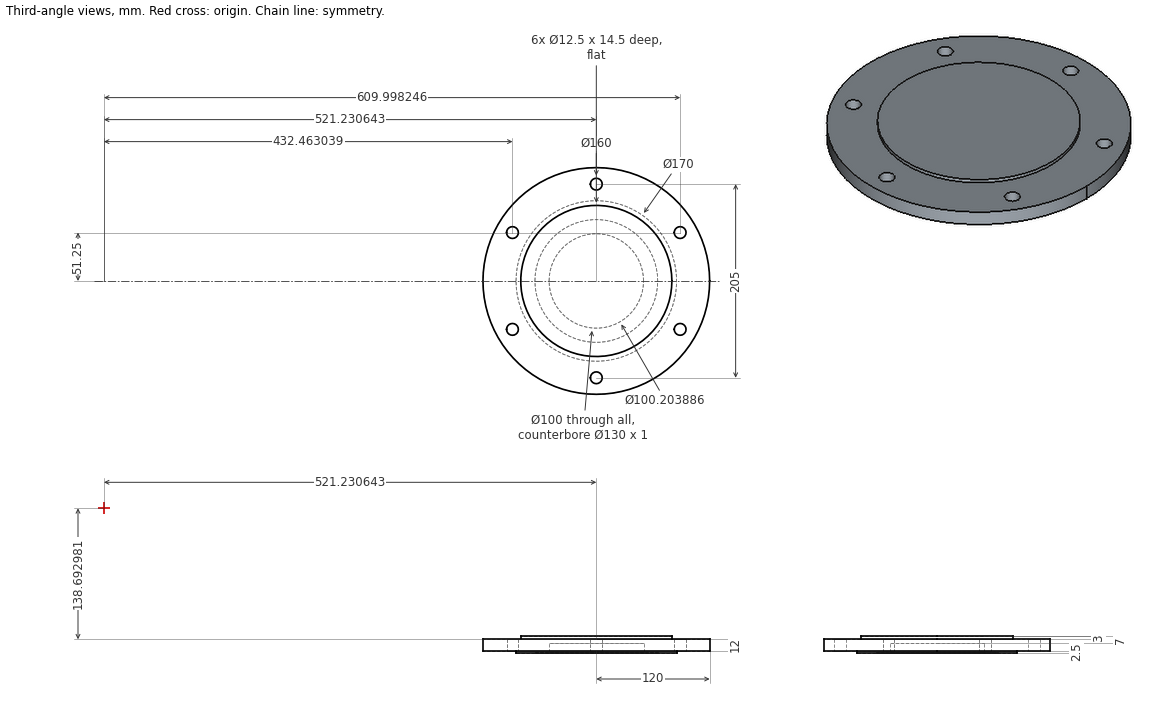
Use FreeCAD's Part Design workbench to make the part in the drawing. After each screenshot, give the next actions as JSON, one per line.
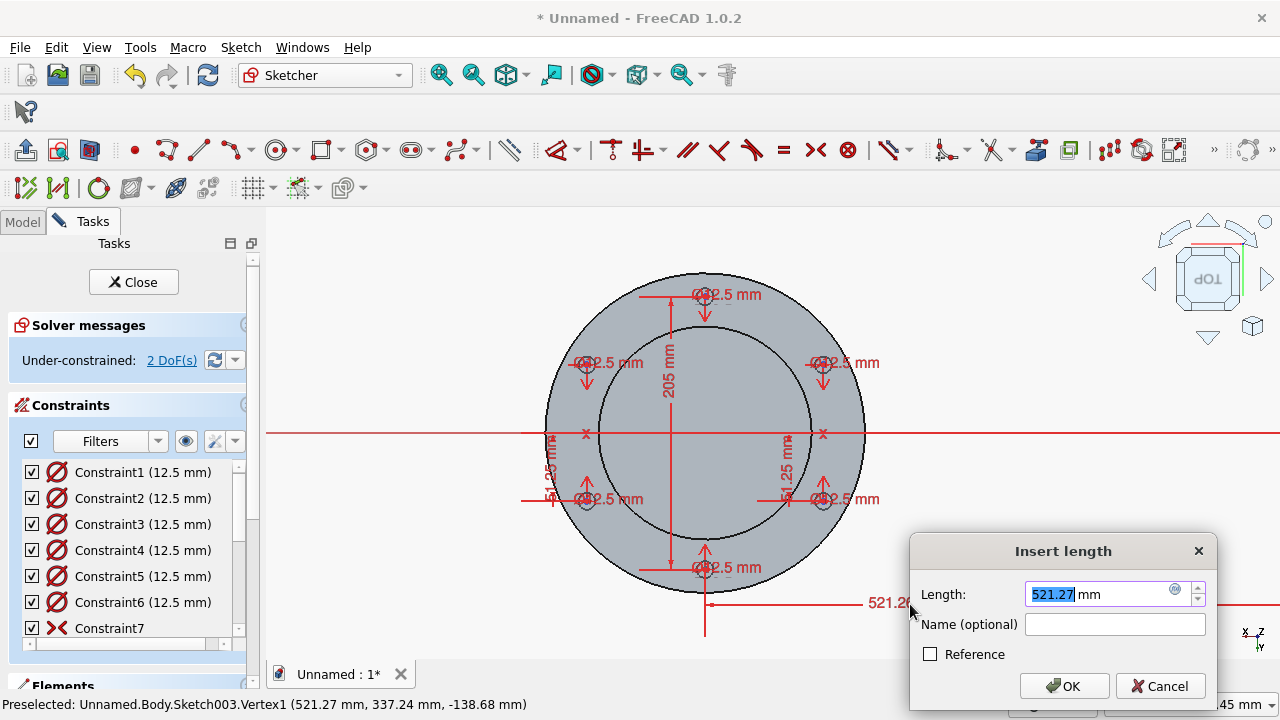
{"action": "type", "text": "521.230643"}
{"action": "key", "text": "Return"}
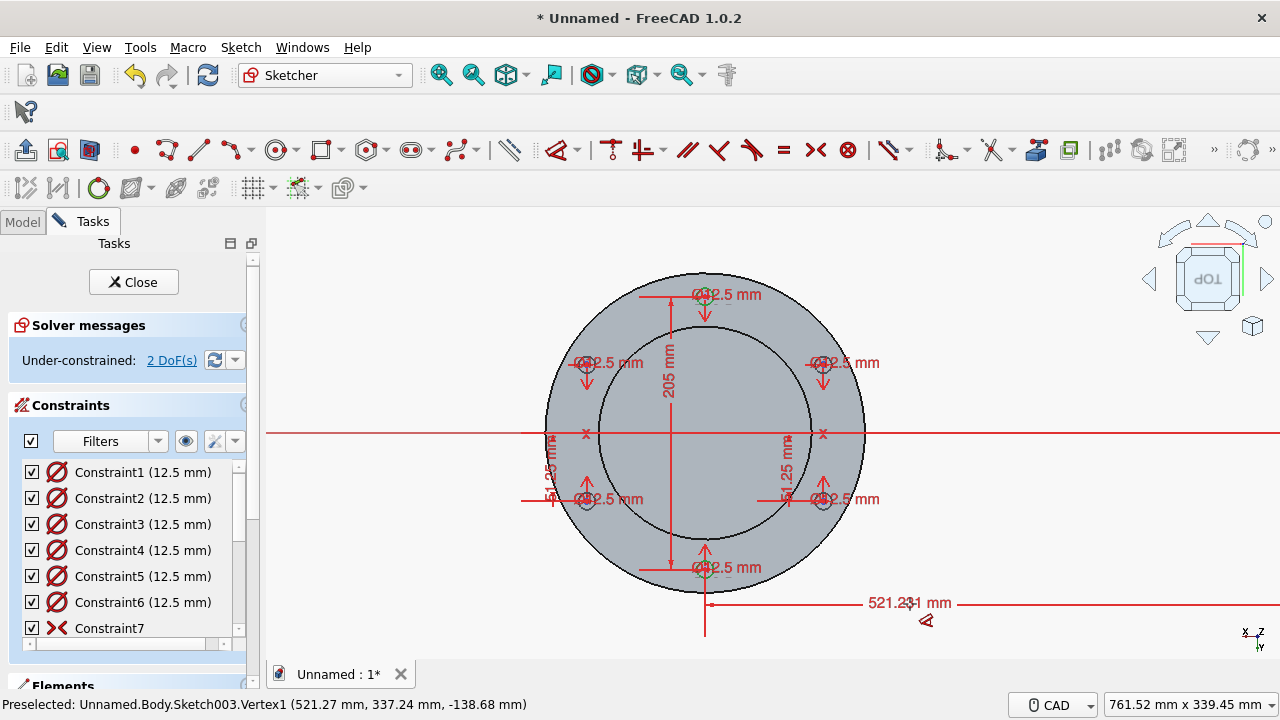
{"action": "left_click", "coordinate": [587, 501]}
{"action": "left_click", "coordinate": [851, 535]}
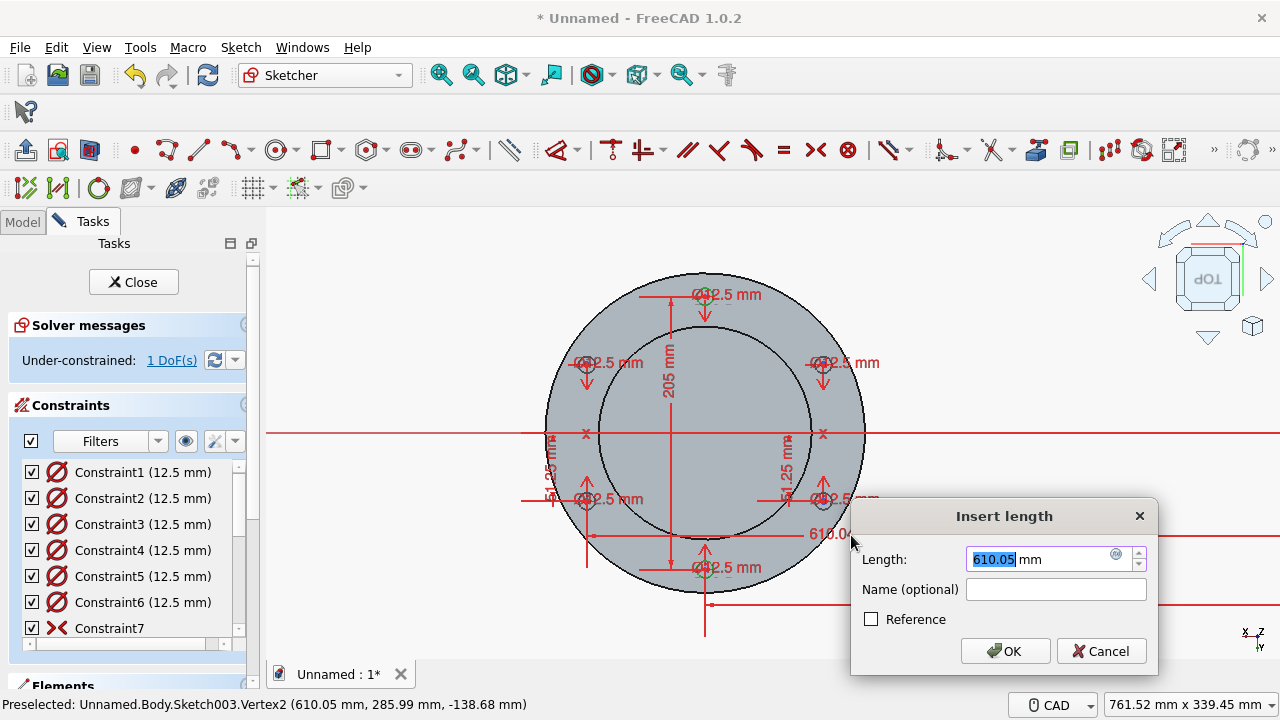
{"action": "type", "text": "609.998246"}
{"action": "key", "text": "Return"}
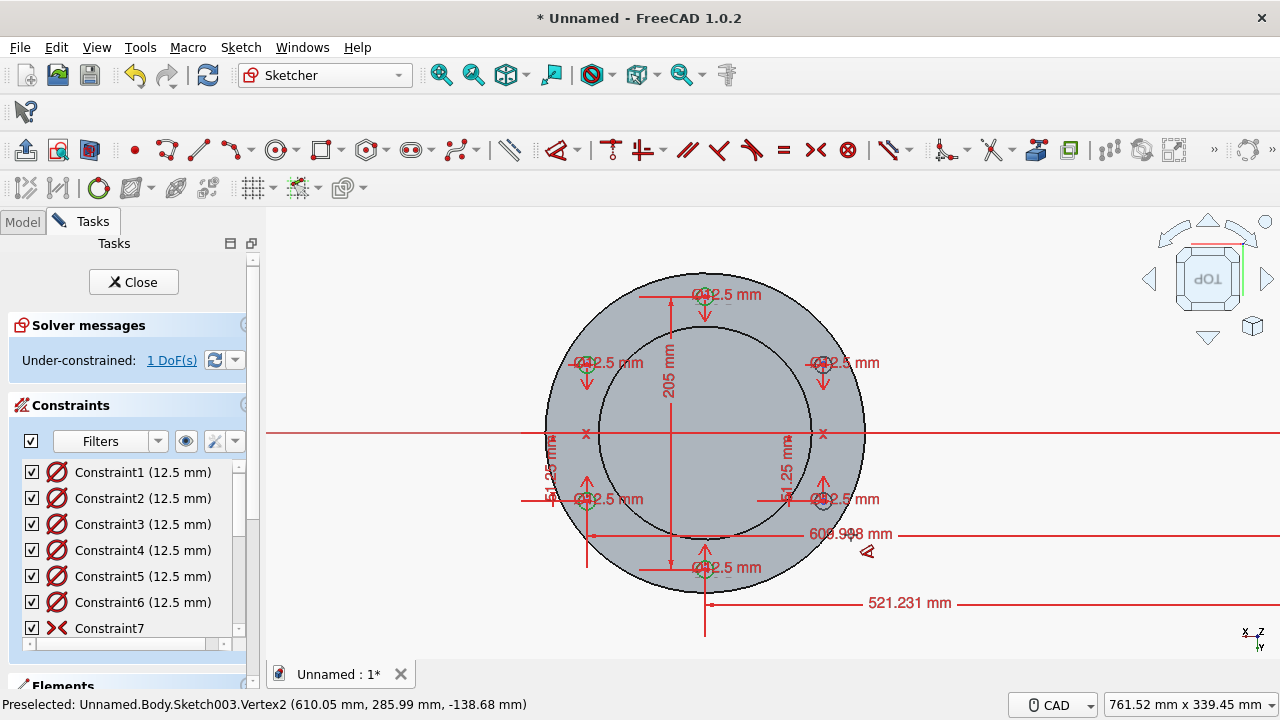
{"action": "left_click", "coordinate": [823, 501]}
{"action": "left_click", "coordinate": [969, 535]}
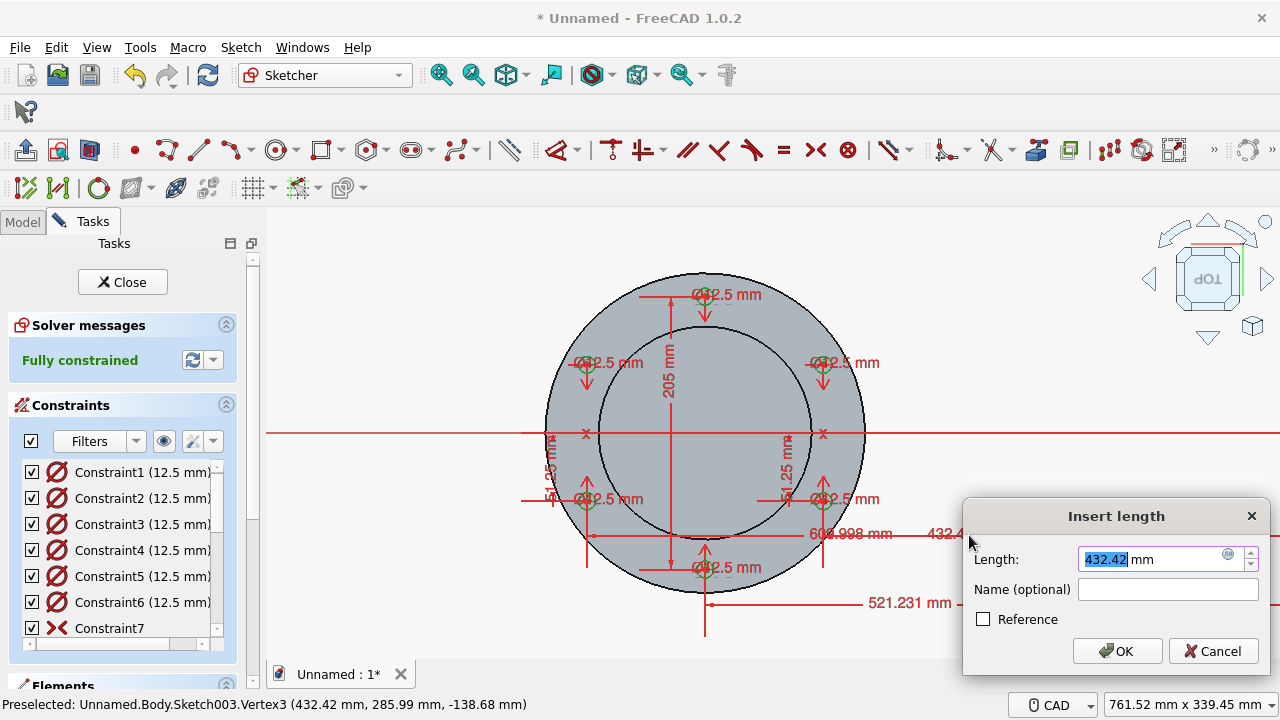
{"action": "type", "text": "432.463039"}
{"action": "key", "text": "Return"}
{"action": "key", "text": "Escape"}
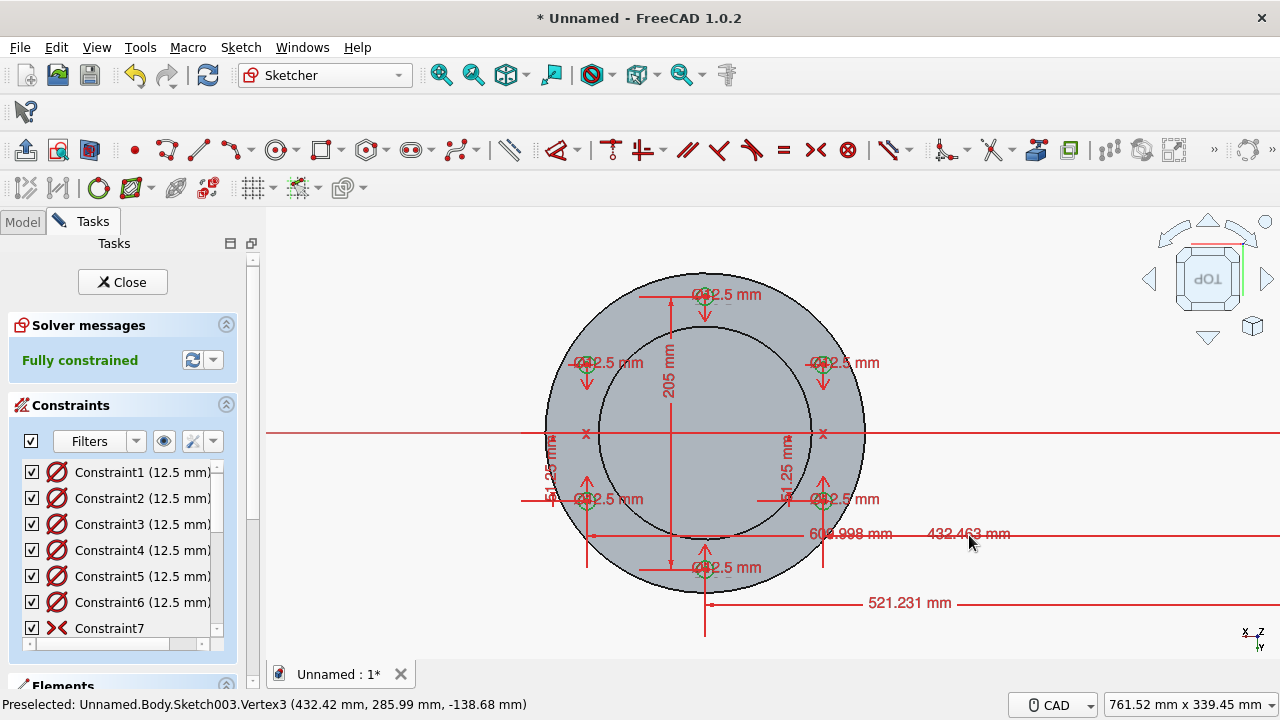
{"action": "left_click", "coordinate": [123, 282]}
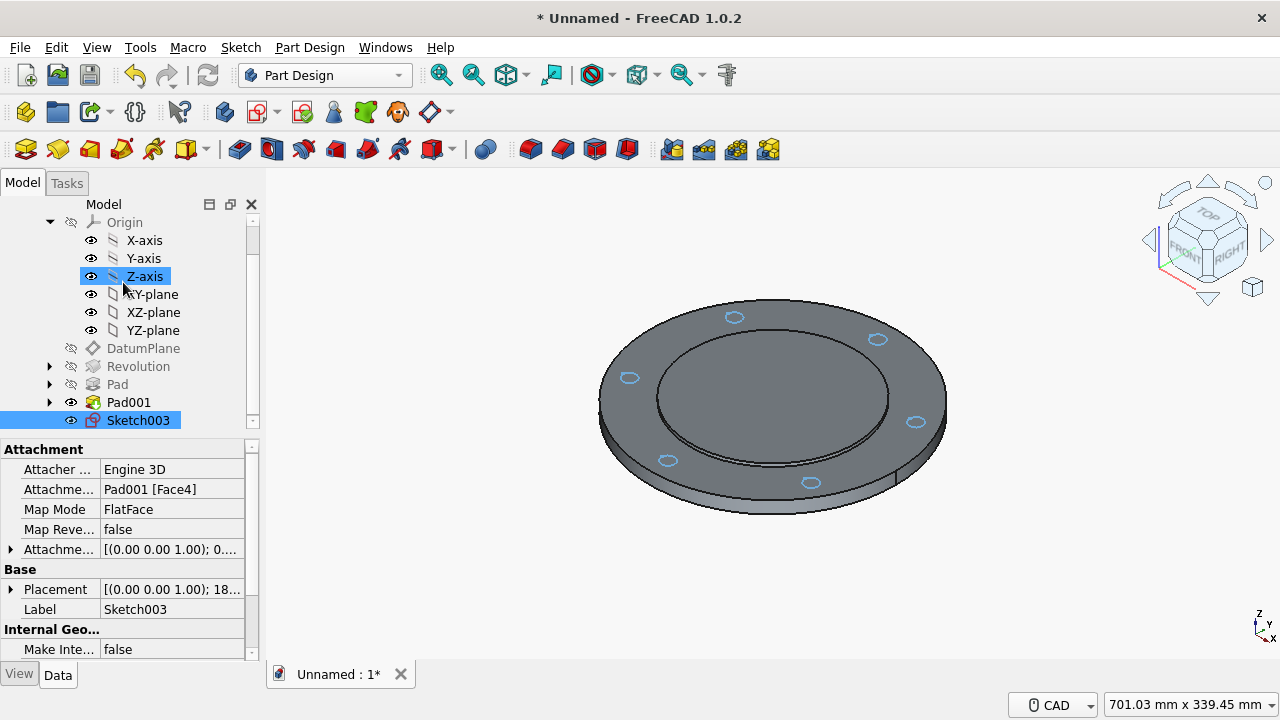
{"action": "left_click", "coordinate": [272, 150]}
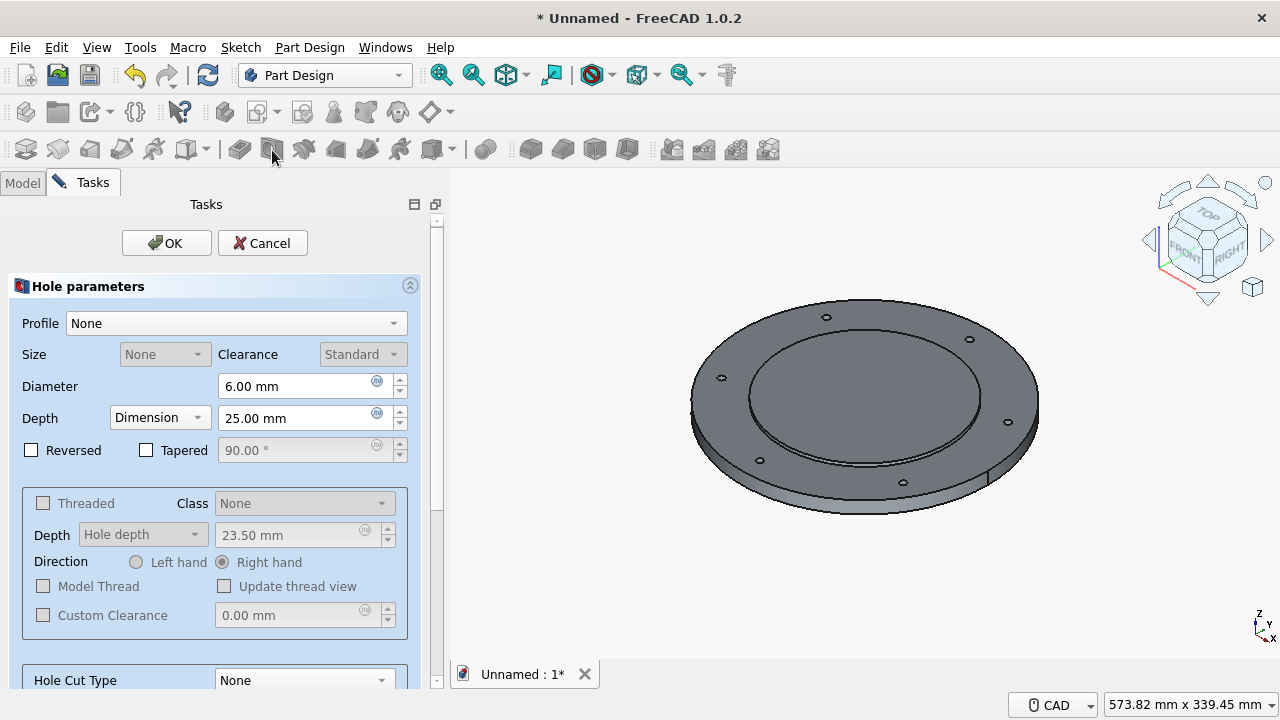
{"action": "triple_click", "coordinate": [305, 386]}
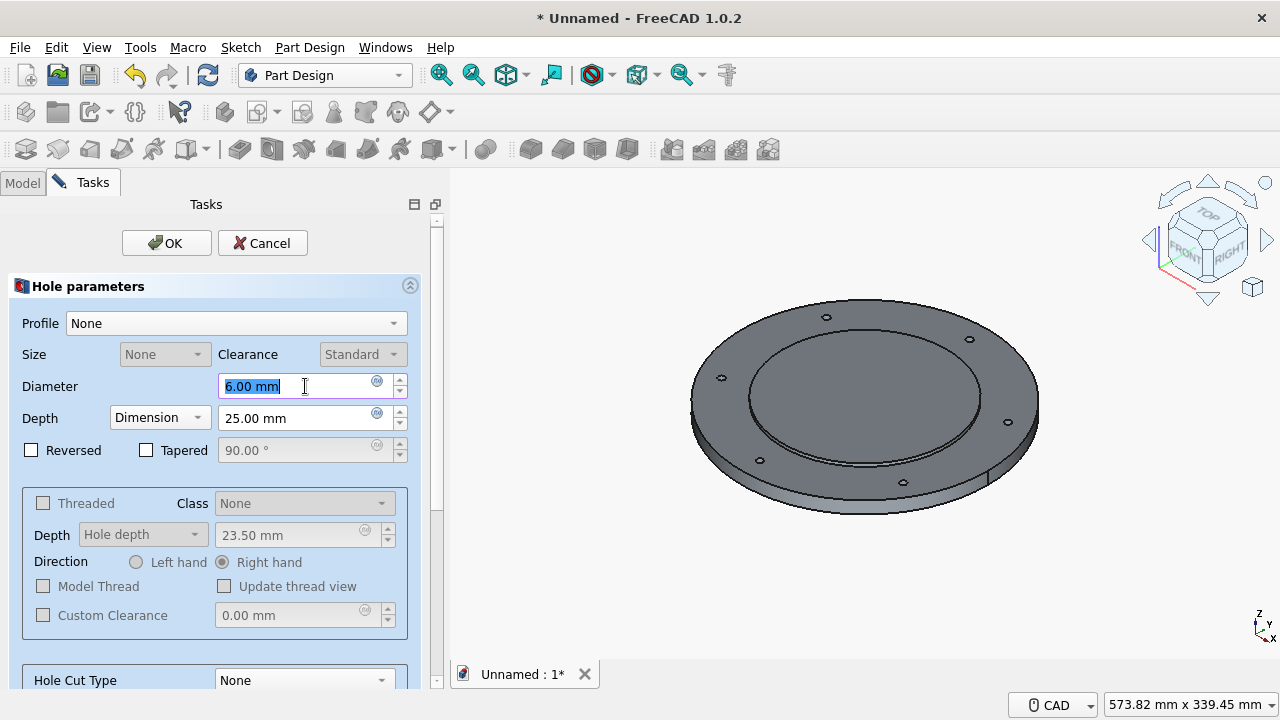
{"action": "type", "text": "12.5"}
{"action": "key", "text": "Tab"}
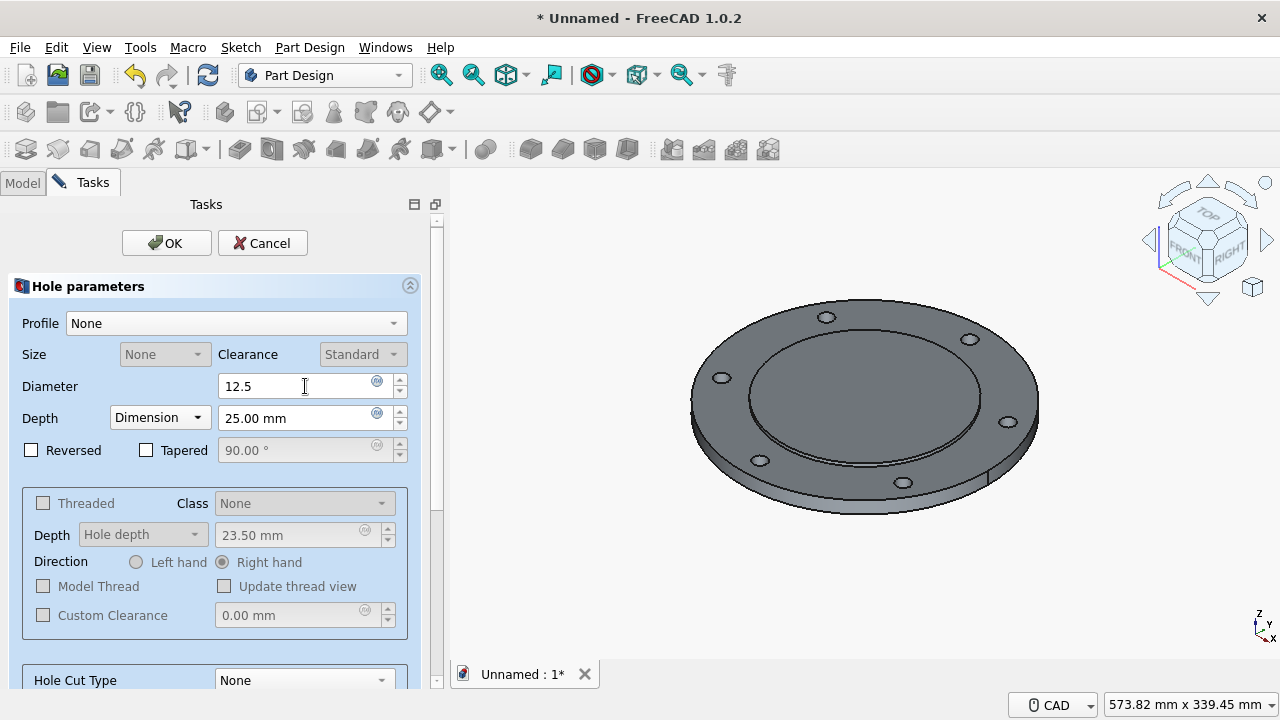
{"action": "triple_click", "coordinate": [305, 418]}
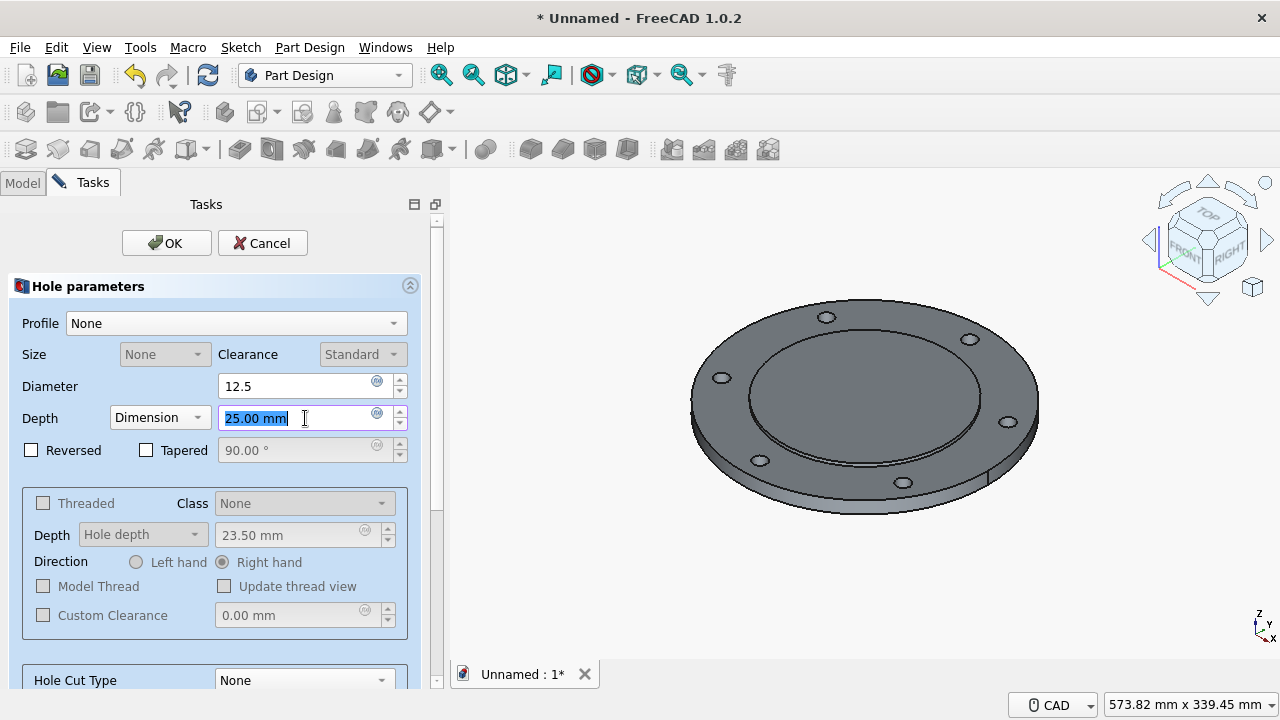
{"action": "type", "text": "14.5"}
{"action": "key", "text": "Tab"}